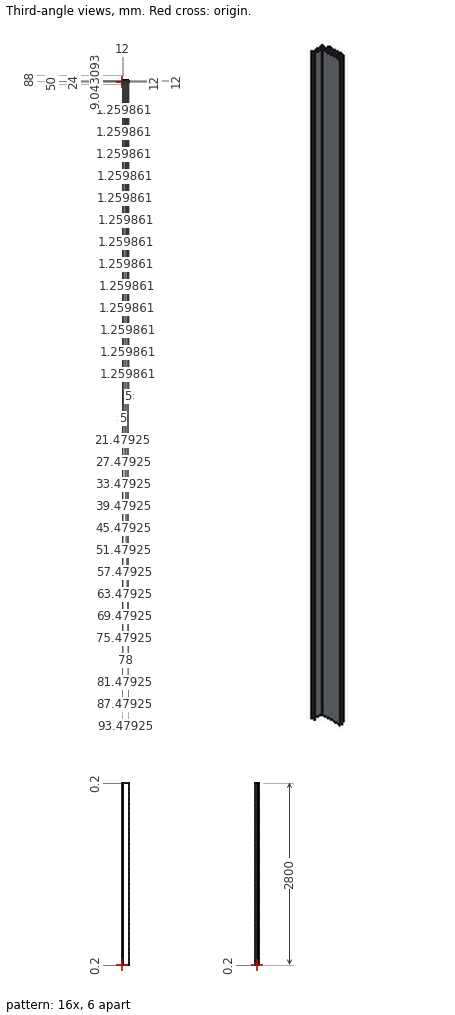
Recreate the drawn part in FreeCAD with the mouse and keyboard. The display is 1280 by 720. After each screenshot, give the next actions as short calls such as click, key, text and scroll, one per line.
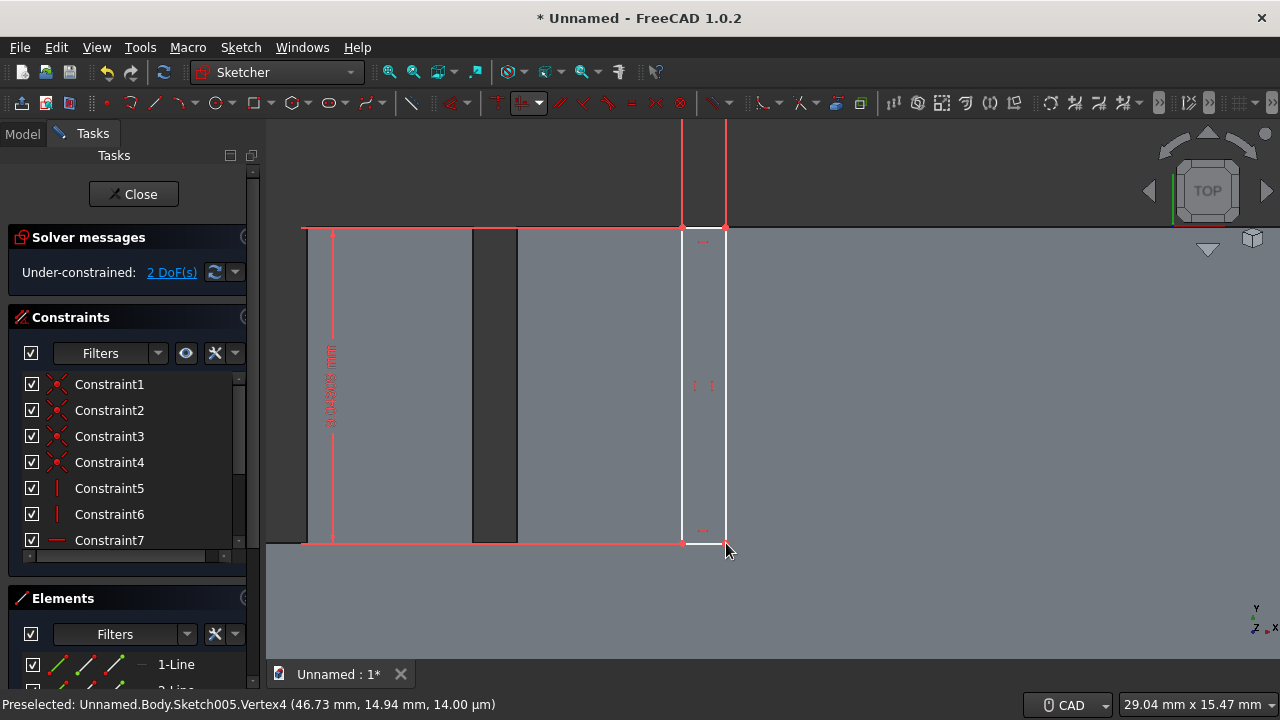
click(450, 104)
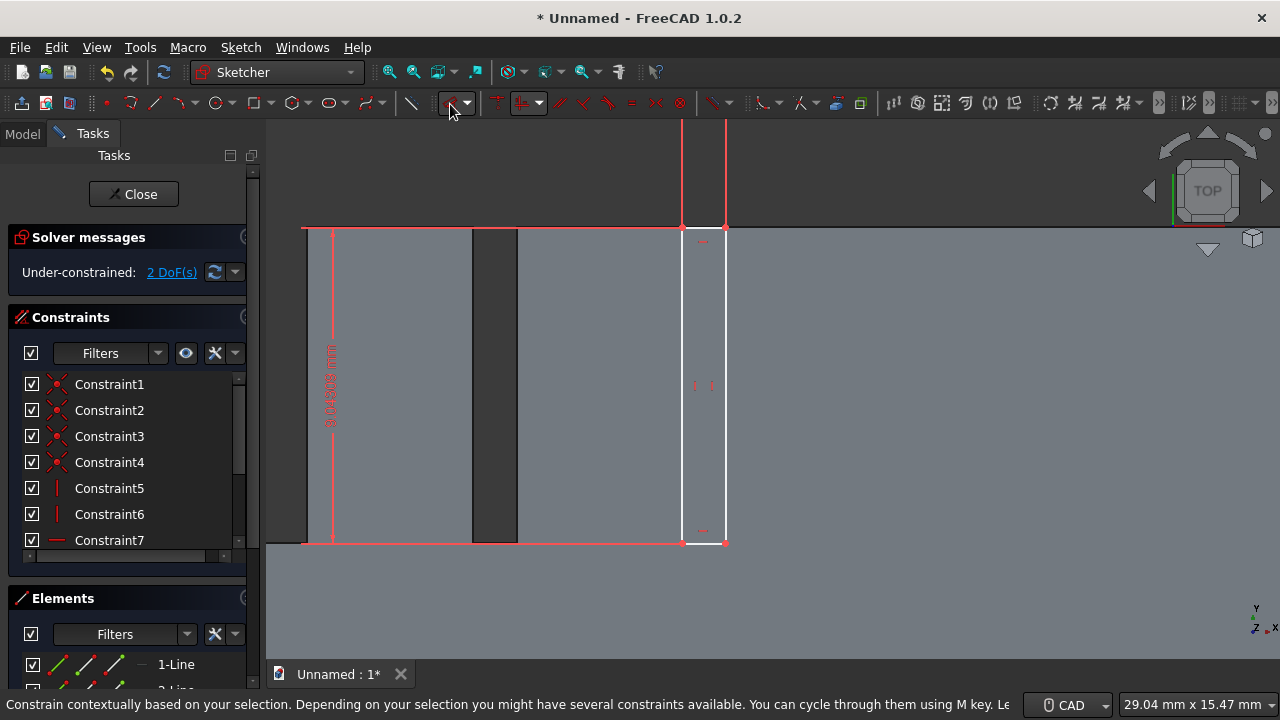
click(682, 228)
click(716, 571)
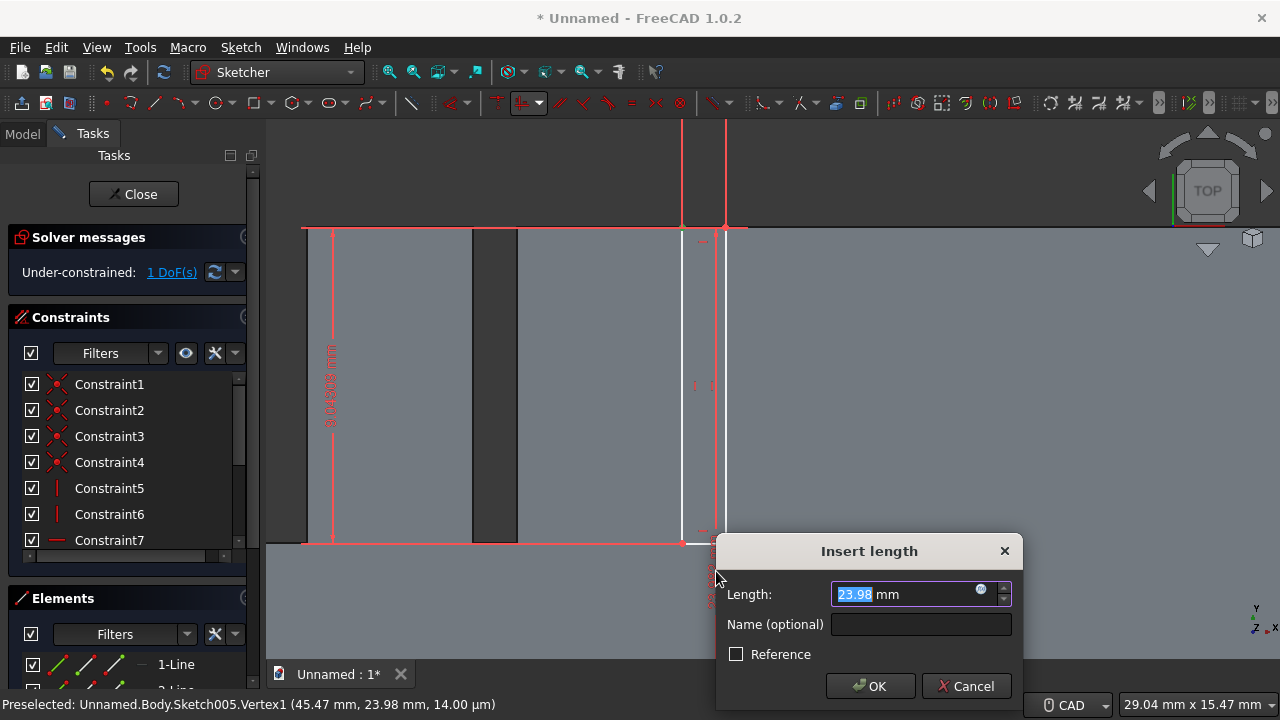
text(24)
key(Return)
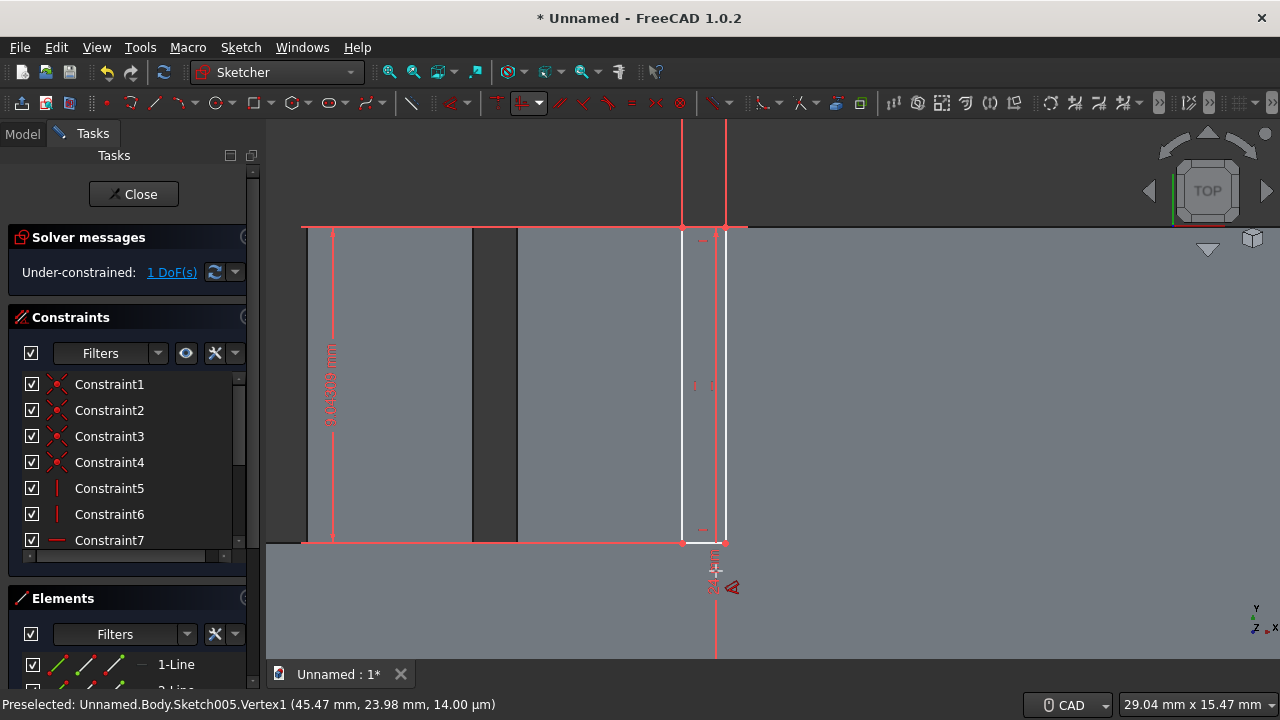
click(682, 227)
click(488, 193)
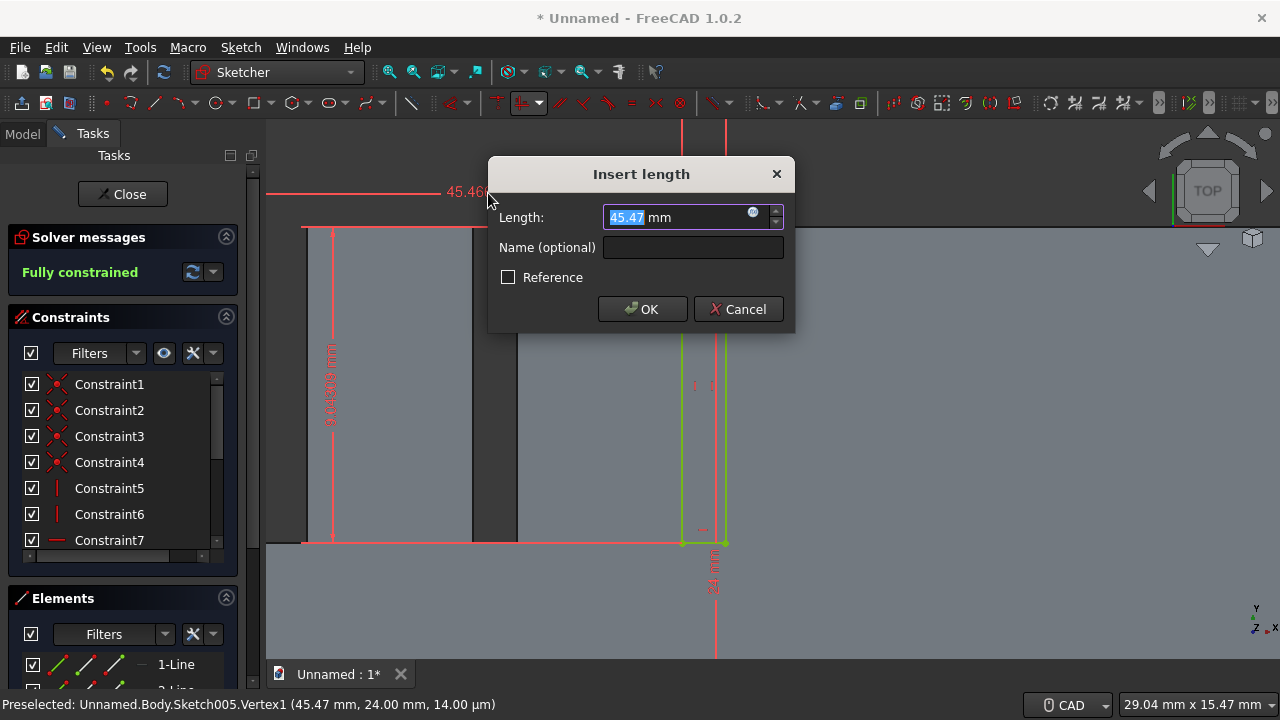
text(45.47925)
key(Return)
key(Escape)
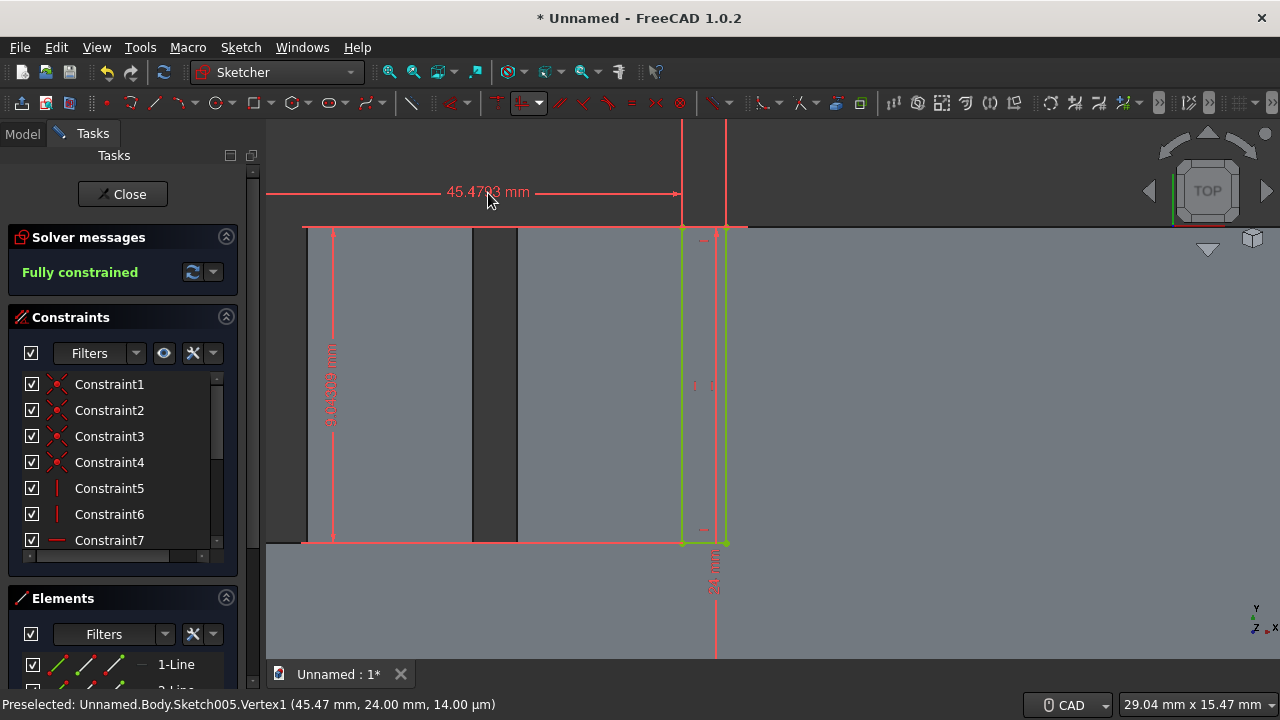
click(123, 194)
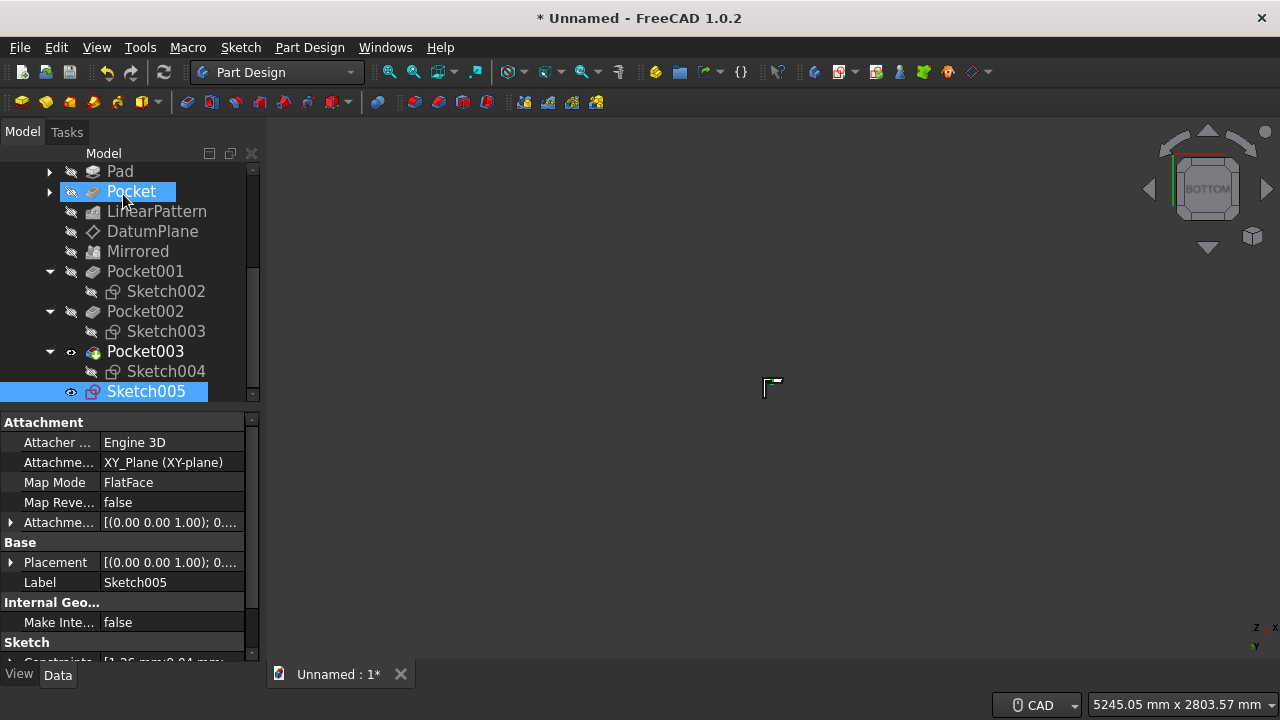
click(188, 102)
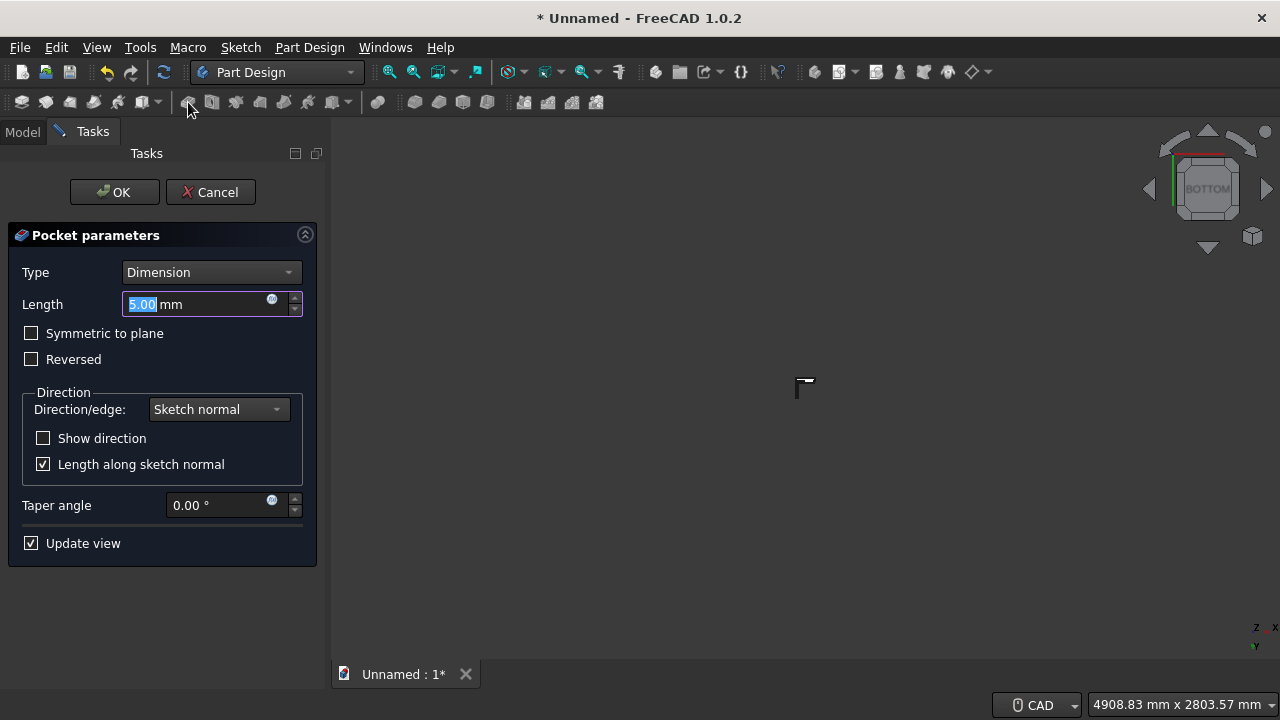
text(0.2)
key(Tab)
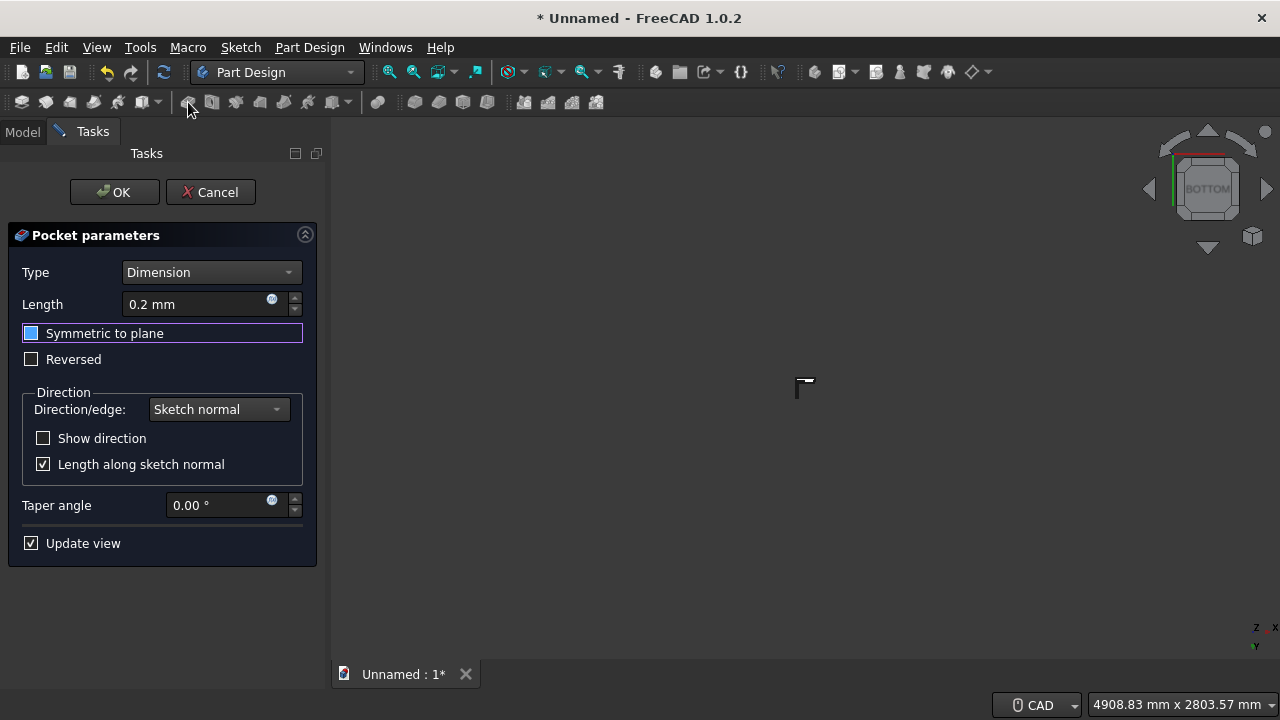
click(30, 359)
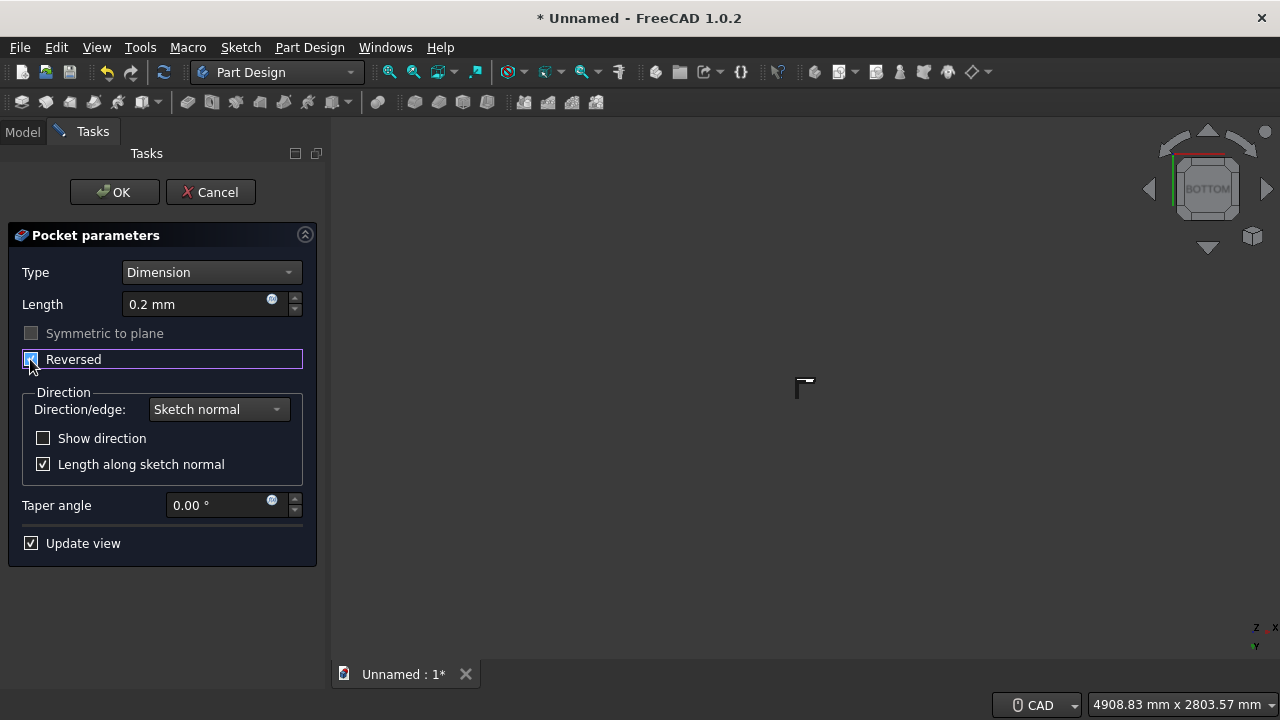
click(115, 192)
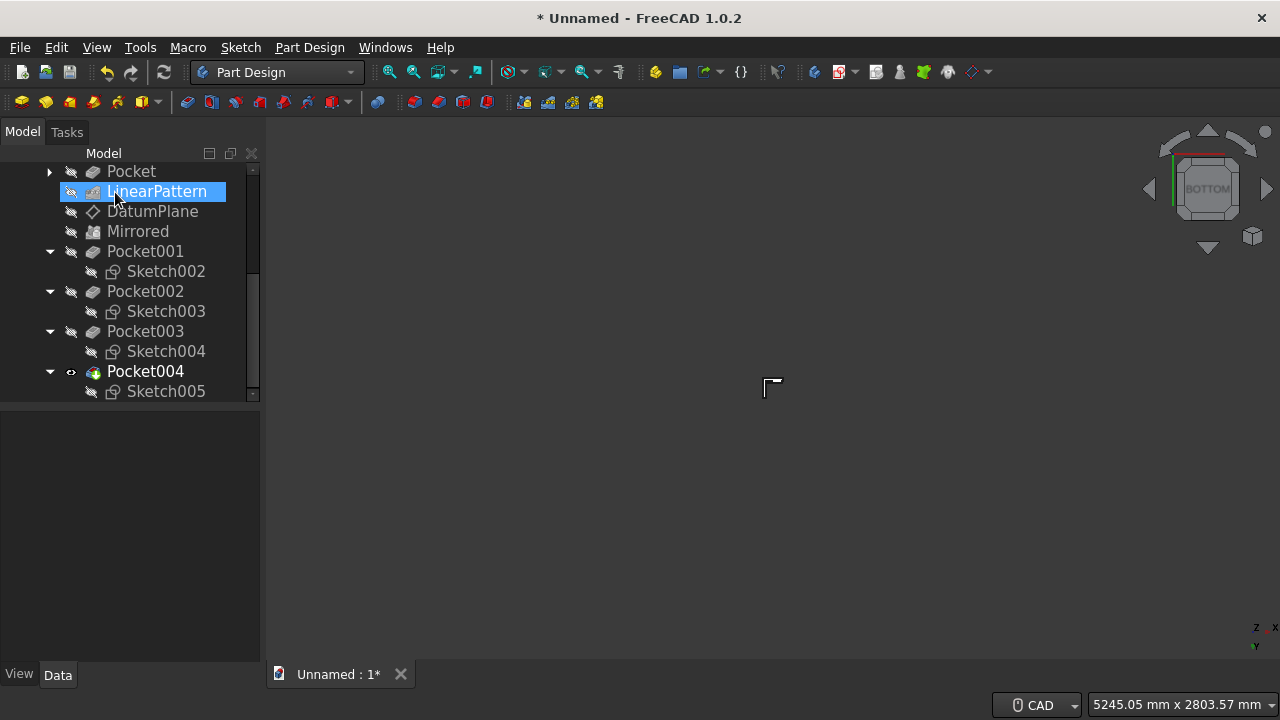
click(390, 72)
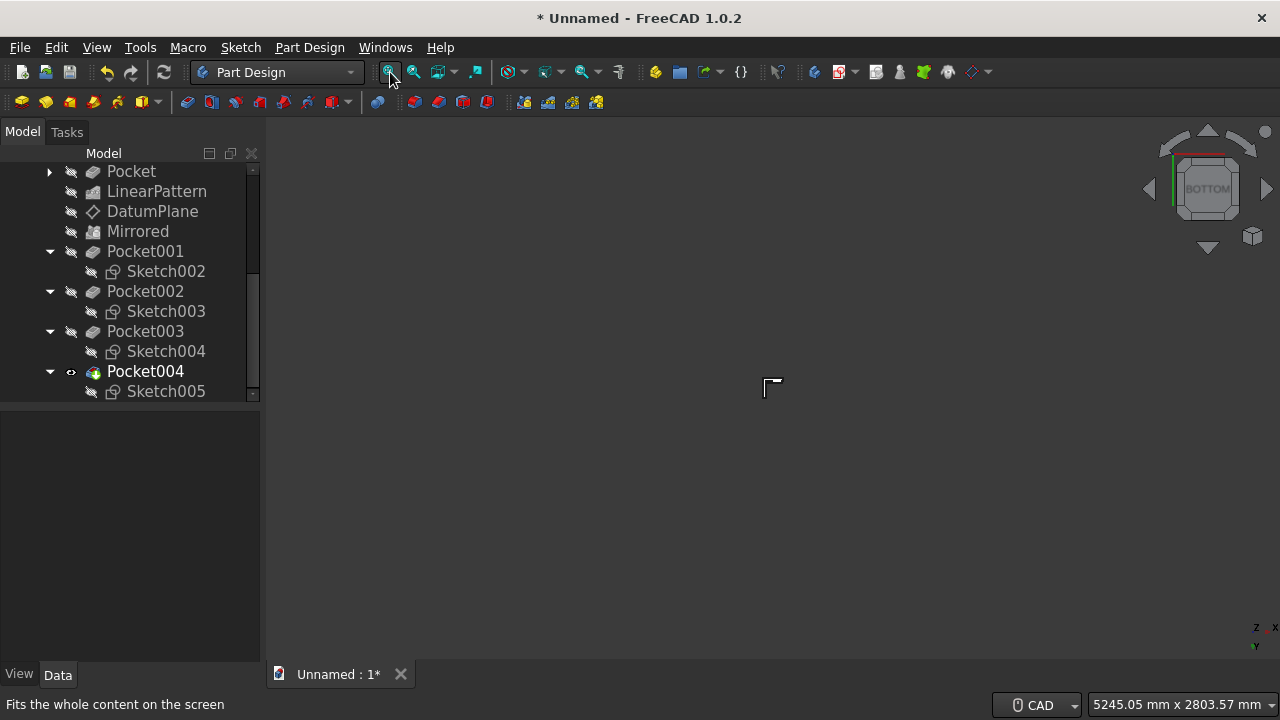
click(840, 72)